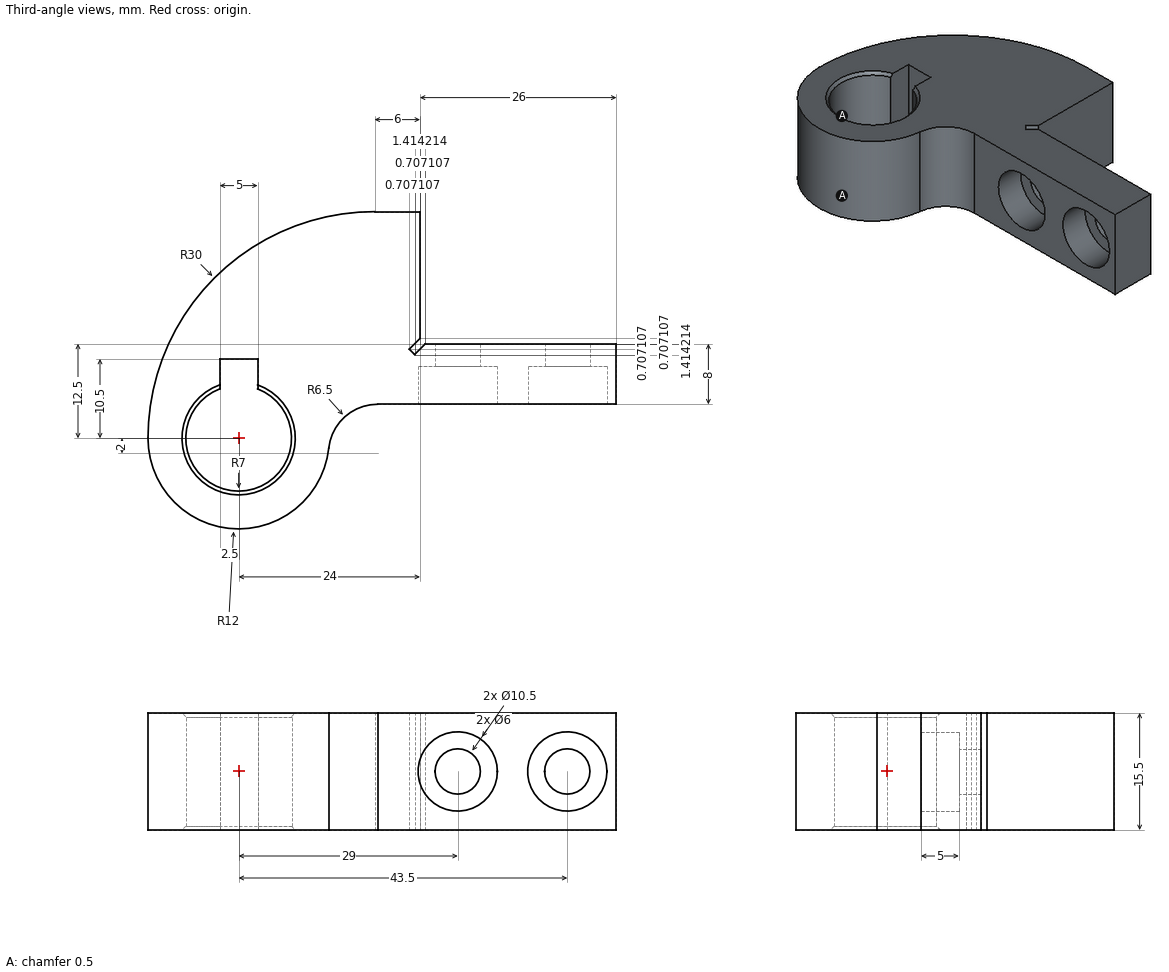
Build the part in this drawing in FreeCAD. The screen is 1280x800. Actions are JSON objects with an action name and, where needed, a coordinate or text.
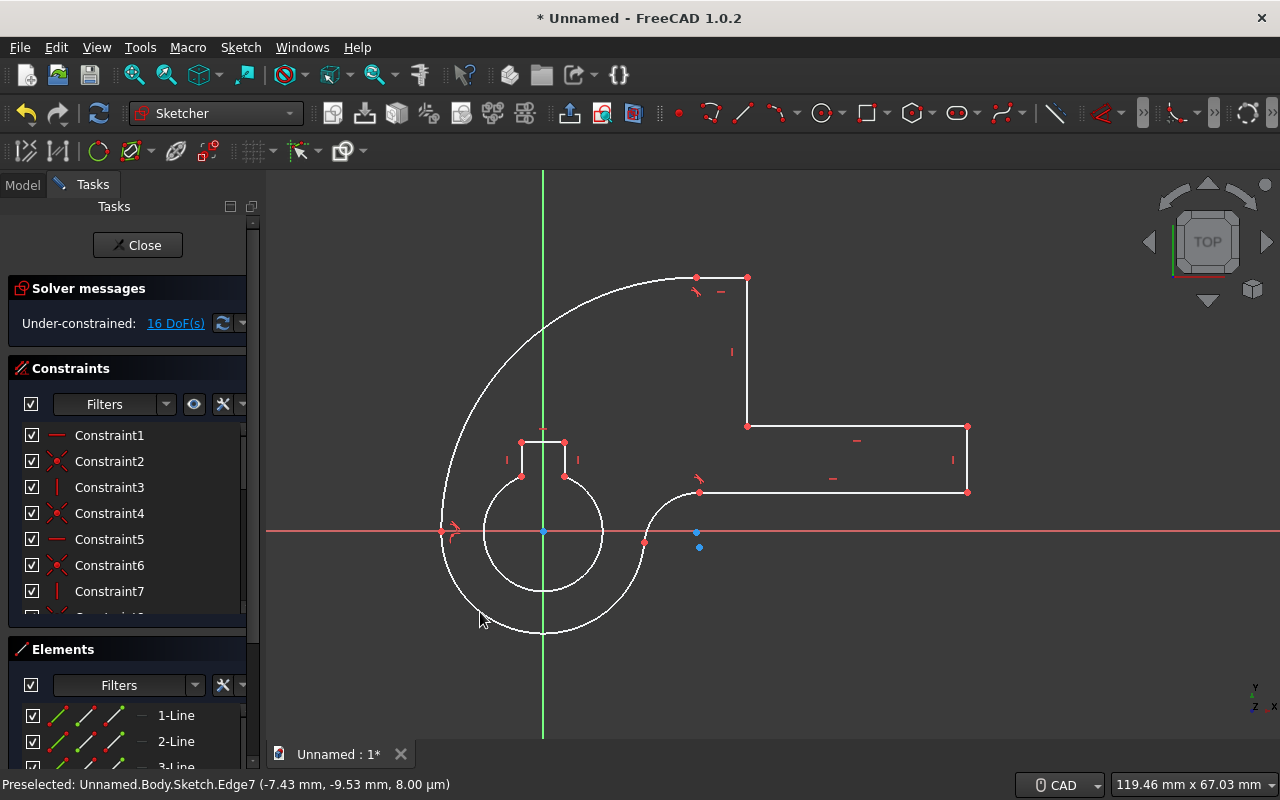
{"action": "left_click", "coordinate": [480, 612]}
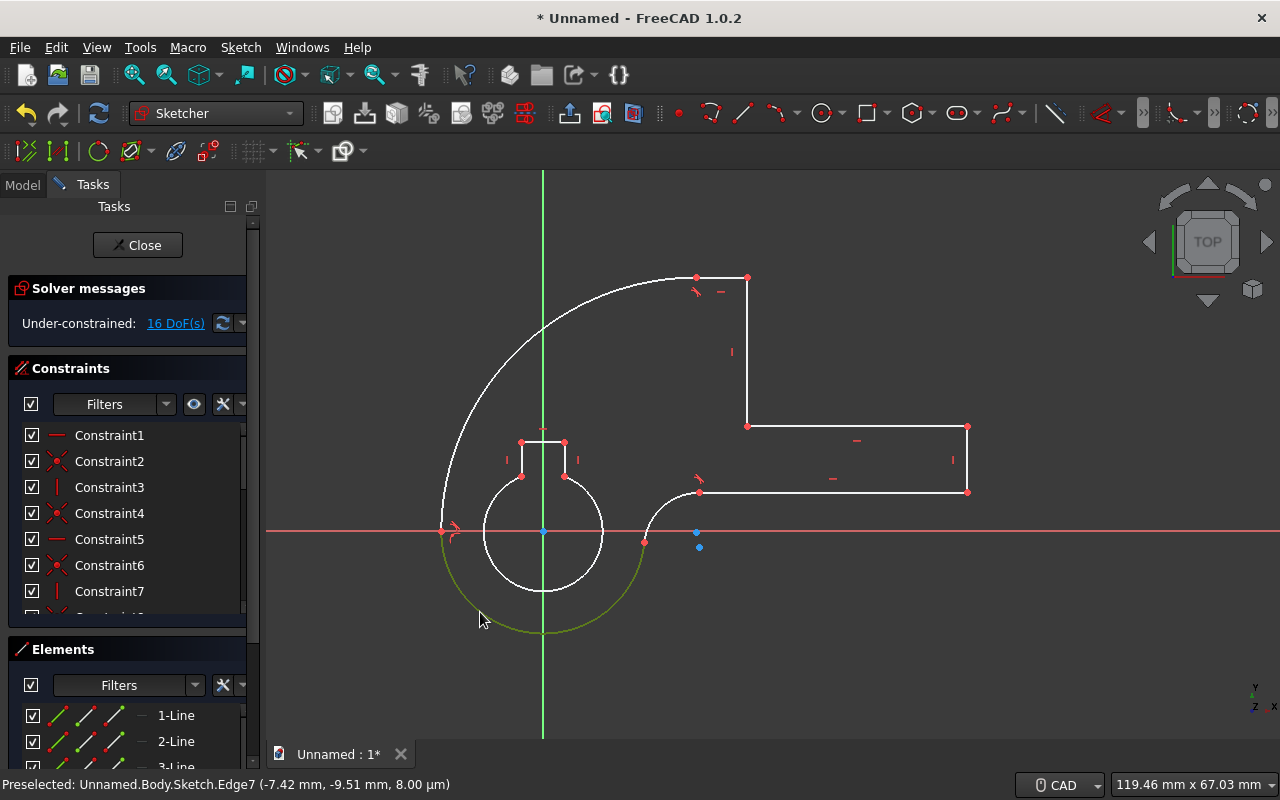
{"action": "left_click", "coordinate": [676, 498]}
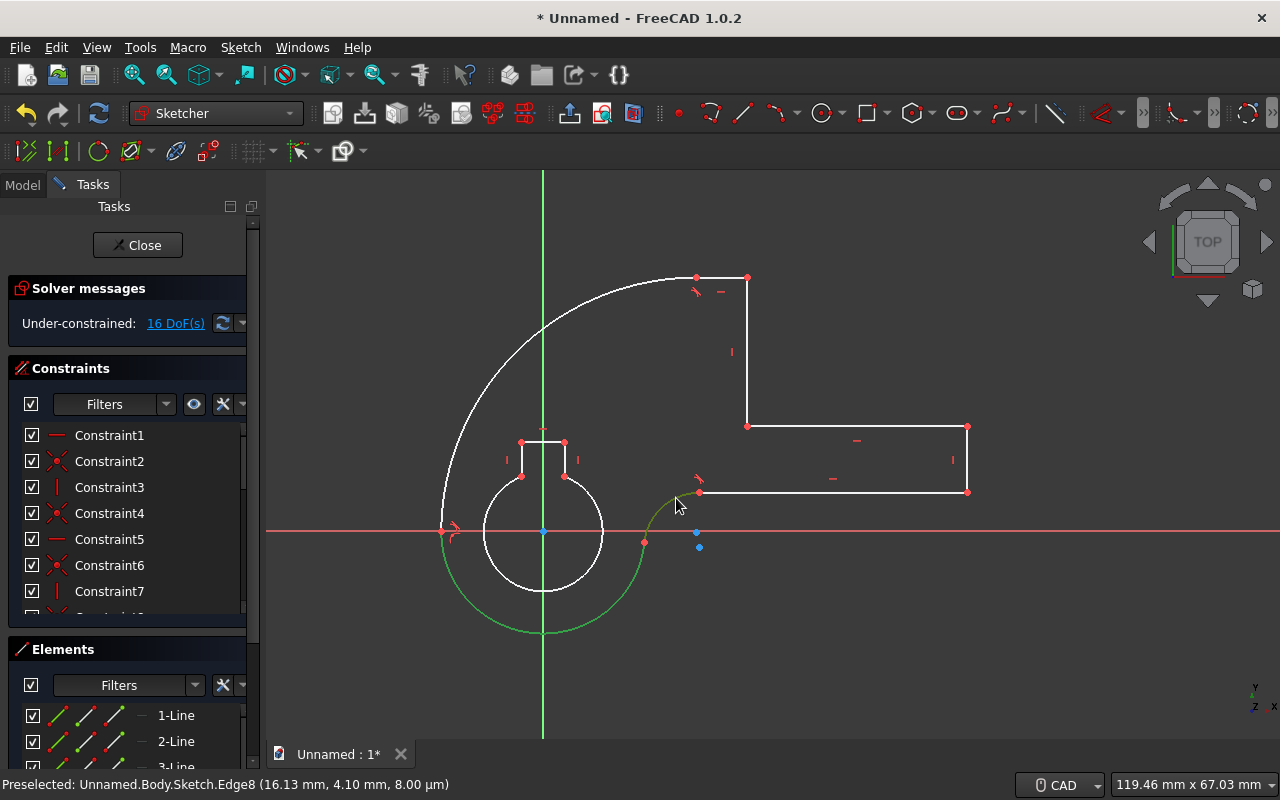
{"action": "key", "text": "t"}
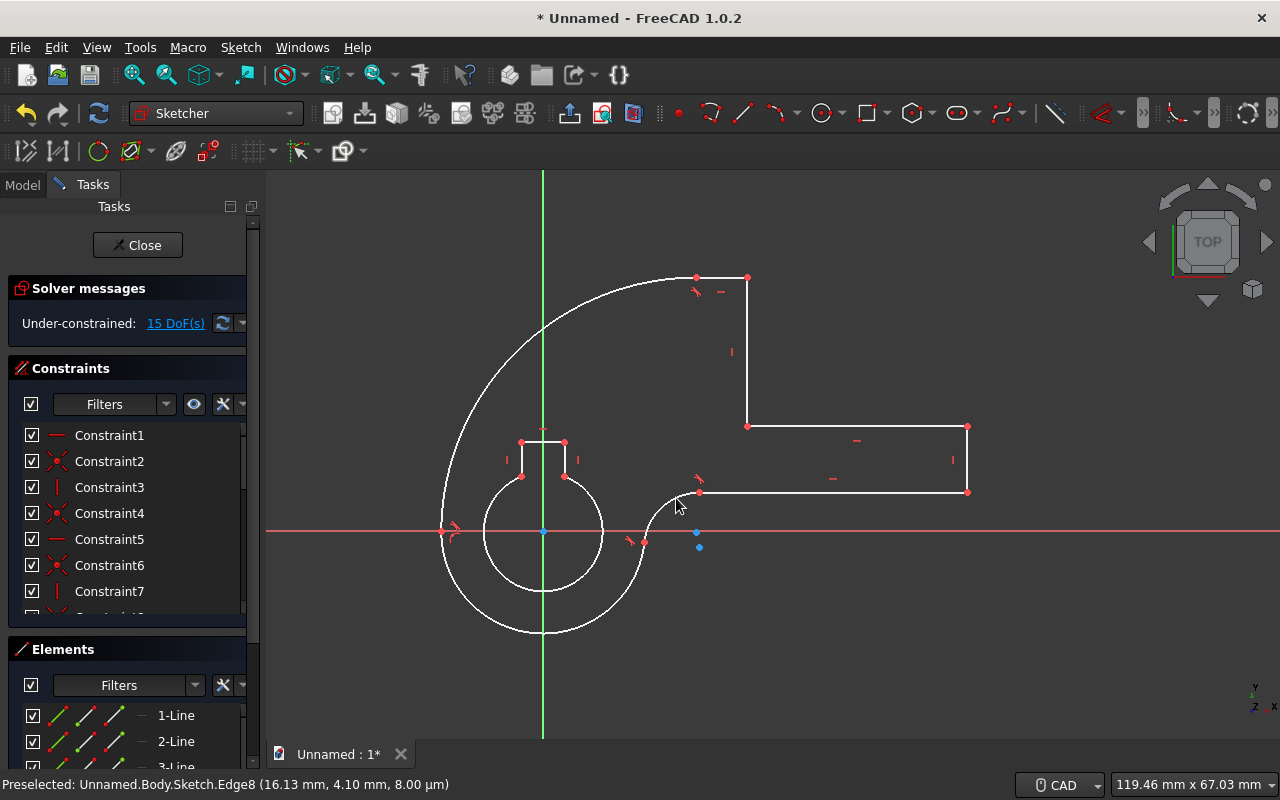
{"action": "left_click", "coordinate": [480, 612]}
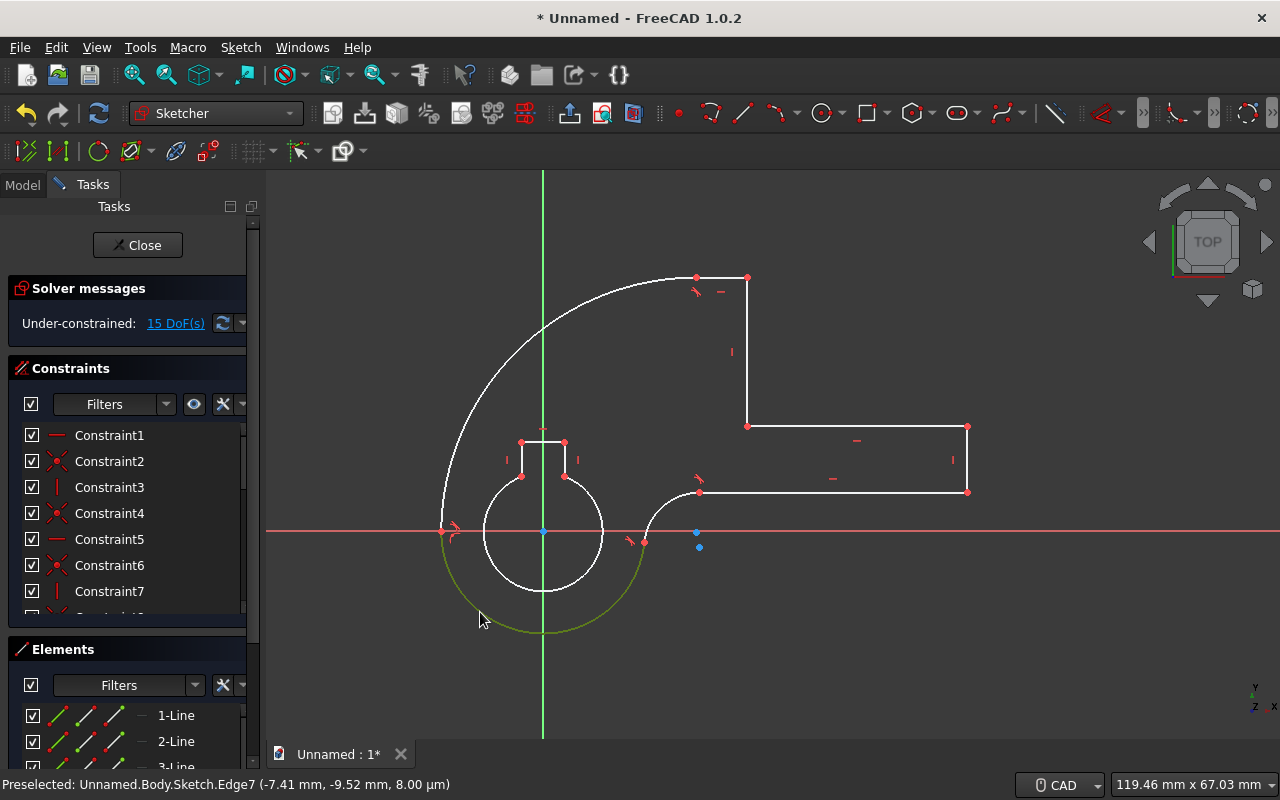
{"action": "left_click", "coordinate": [490, 558]}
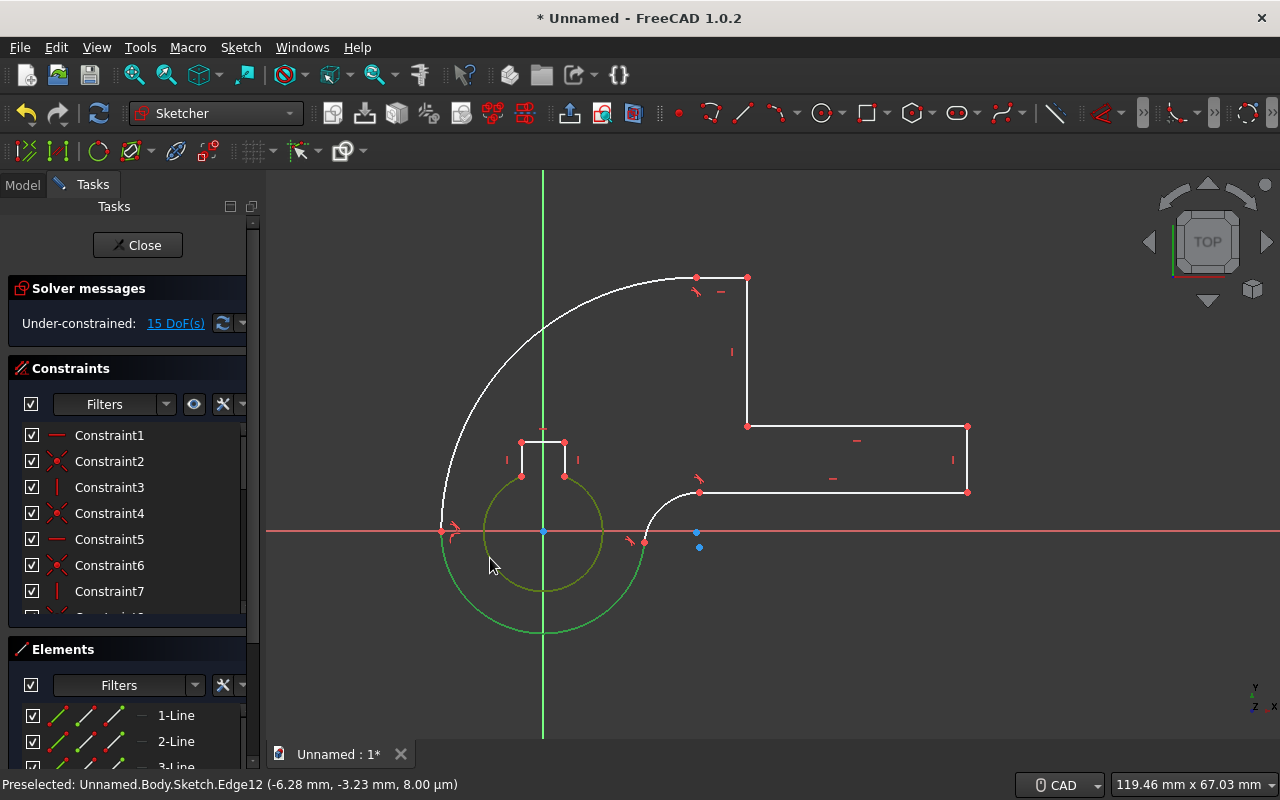
{"action": "key", "text": "c"}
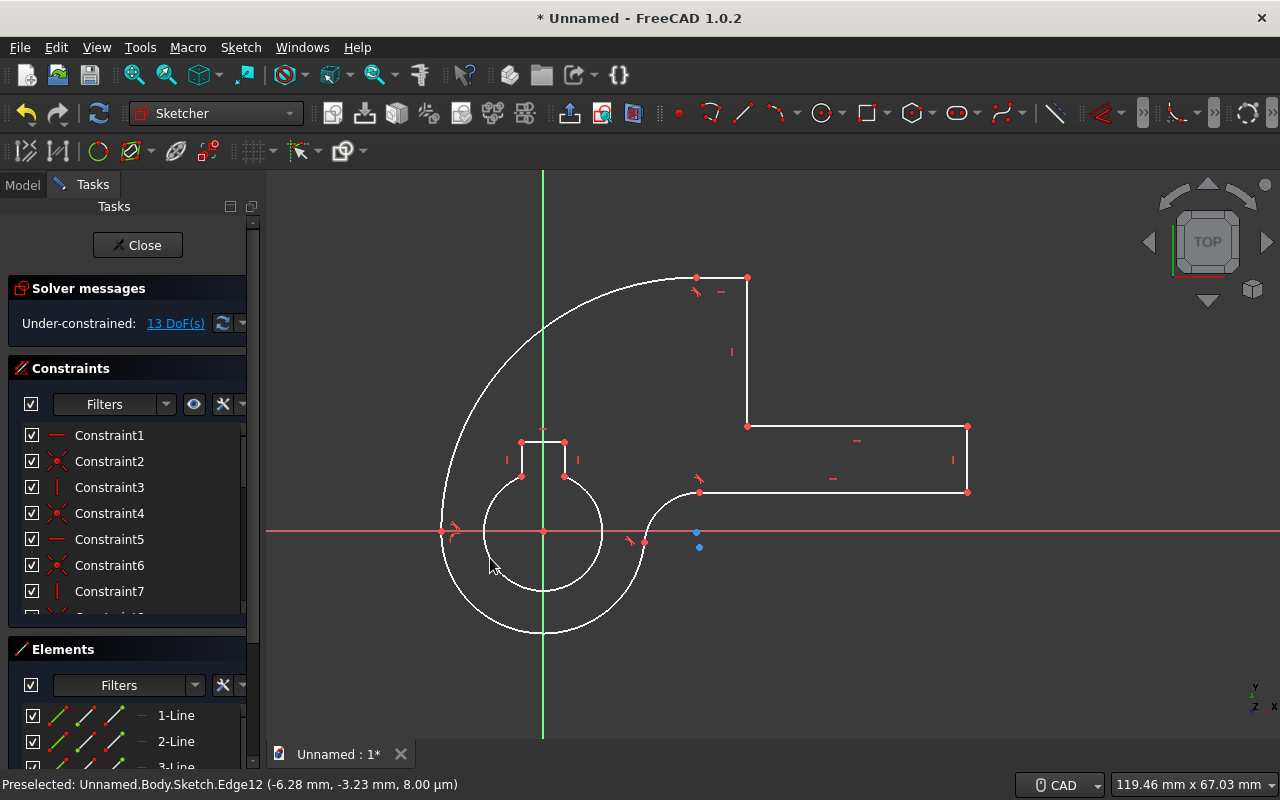
{"action": "left_click_drag", "start_coordinate": [533, 521], "coordinate": [553, 542]}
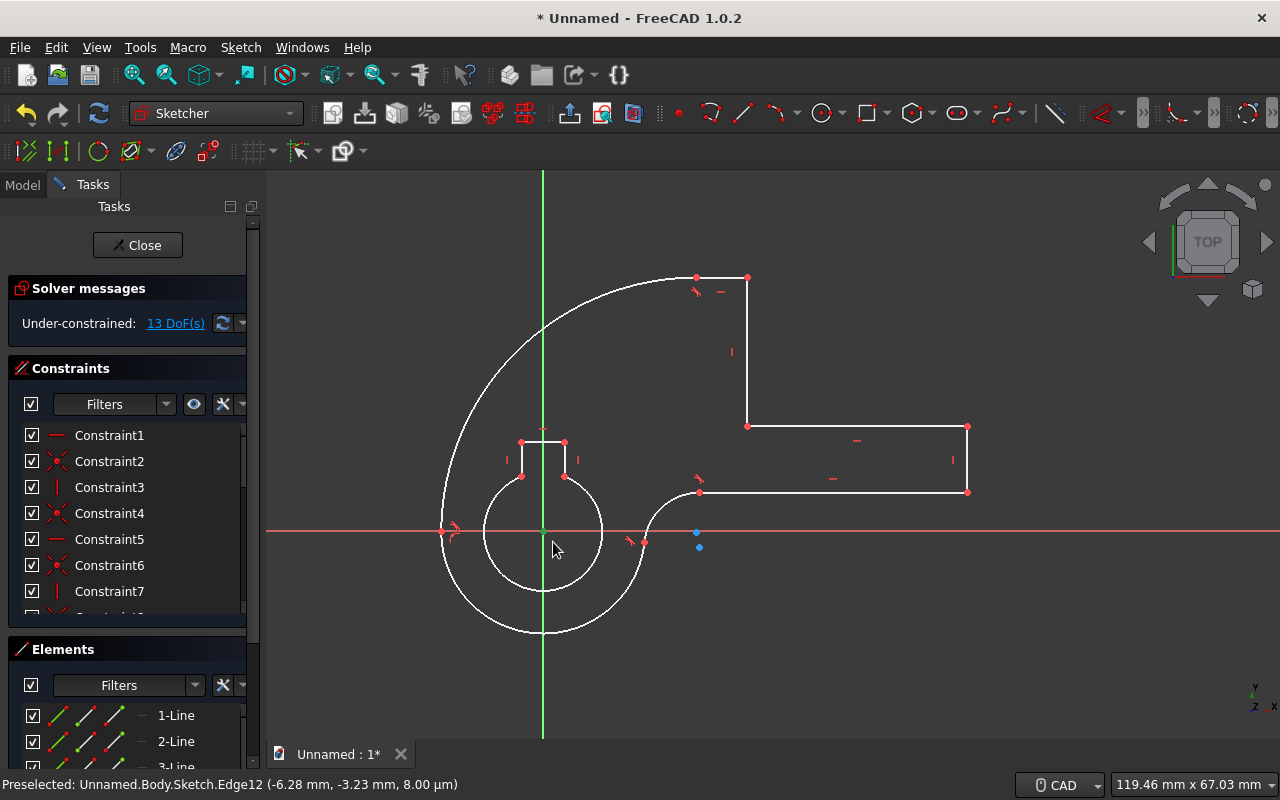
{"action": "key", "text": "c"}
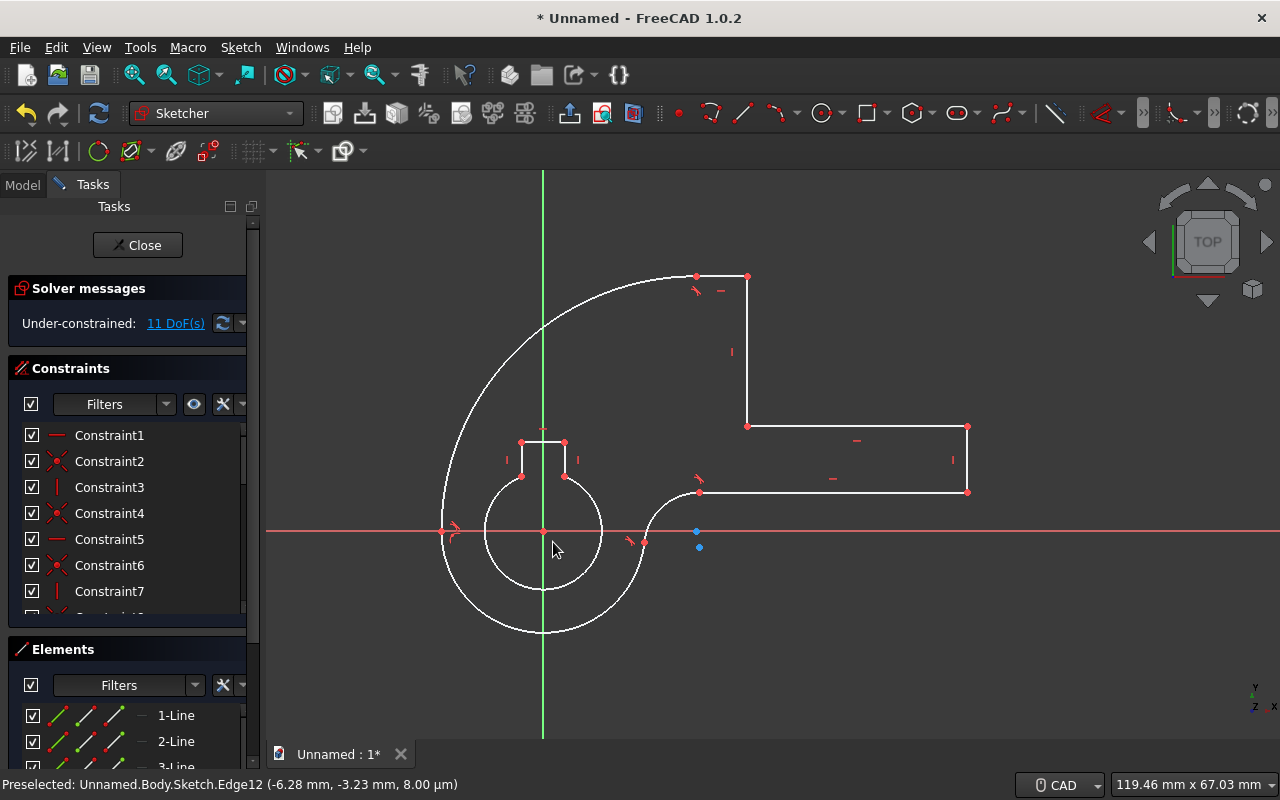
{"action": "key", "text": "d"}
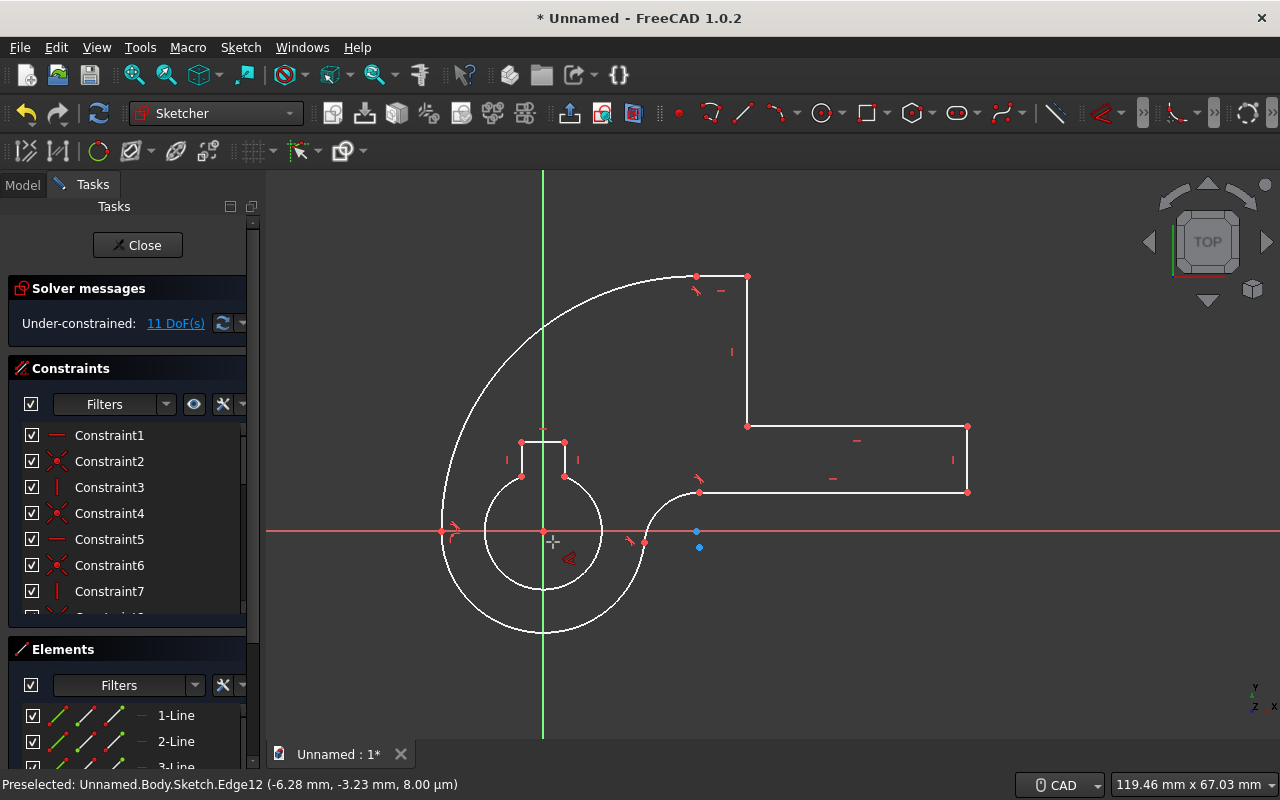
{"action": "left_click", "coordinate": [581, 304]}
{"action": "left_click", "coordinate": [567, 275]}